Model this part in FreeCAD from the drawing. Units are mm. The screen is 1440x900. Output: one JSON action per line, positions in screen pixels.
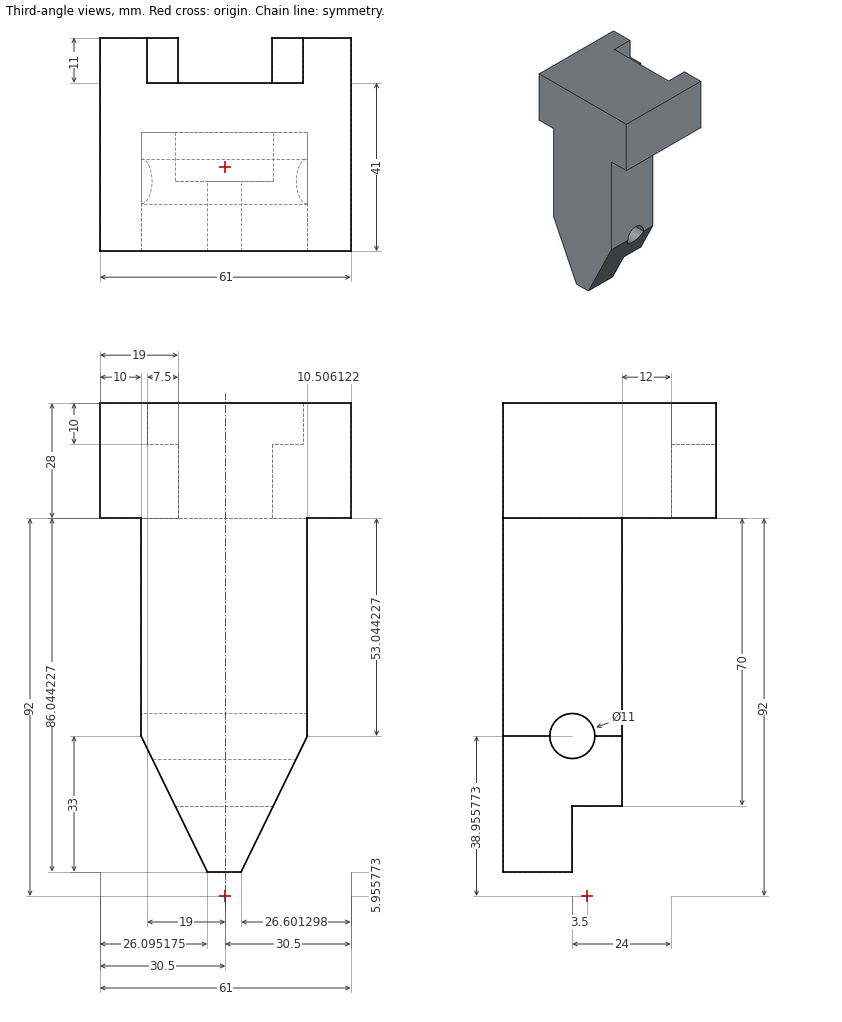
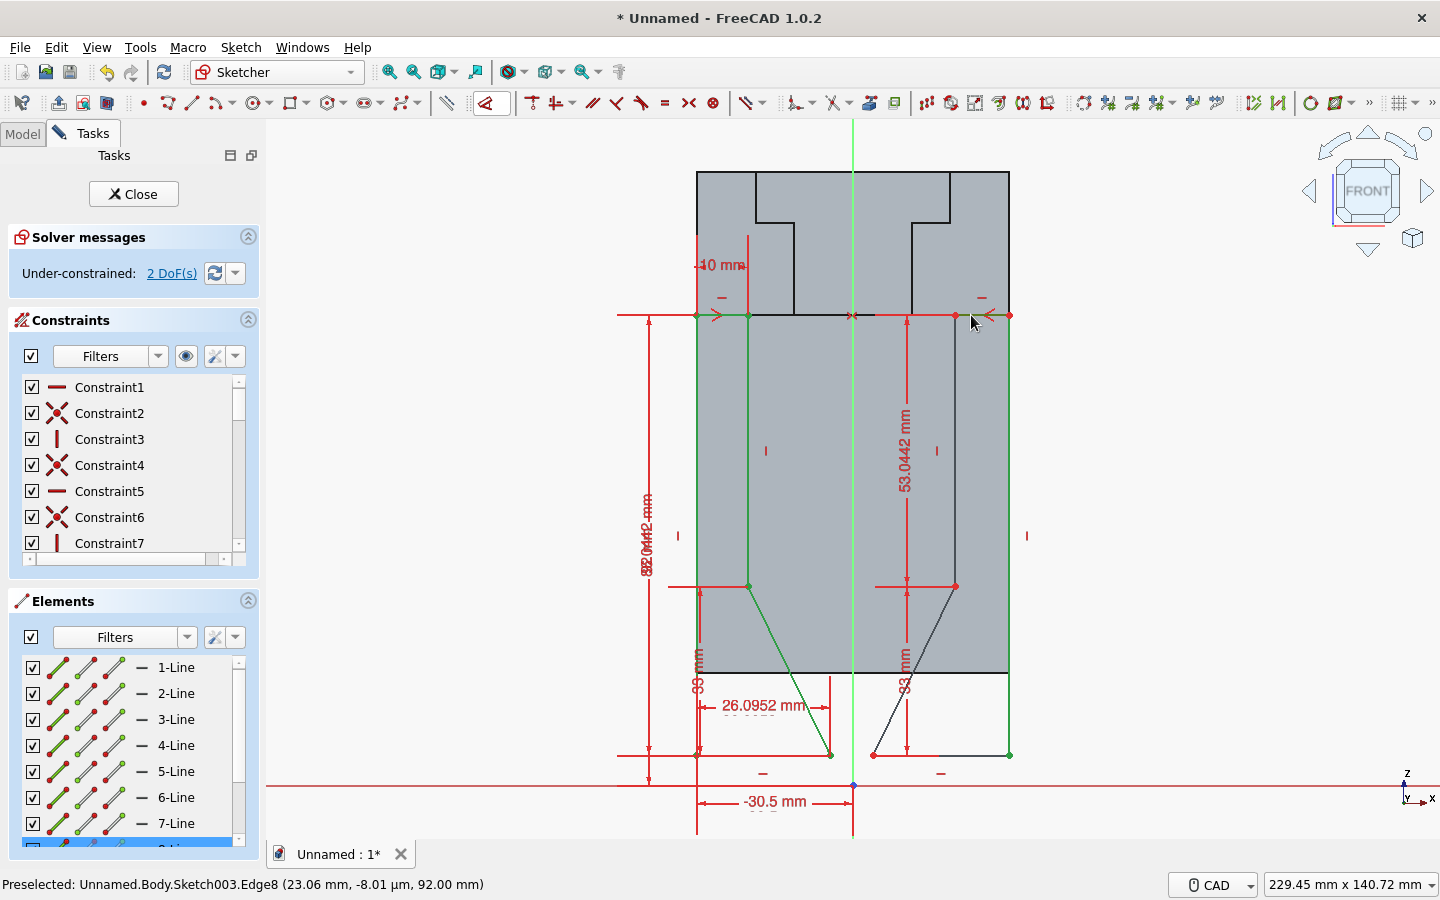
{"action": "left_click", "coordinate": [504, 104]}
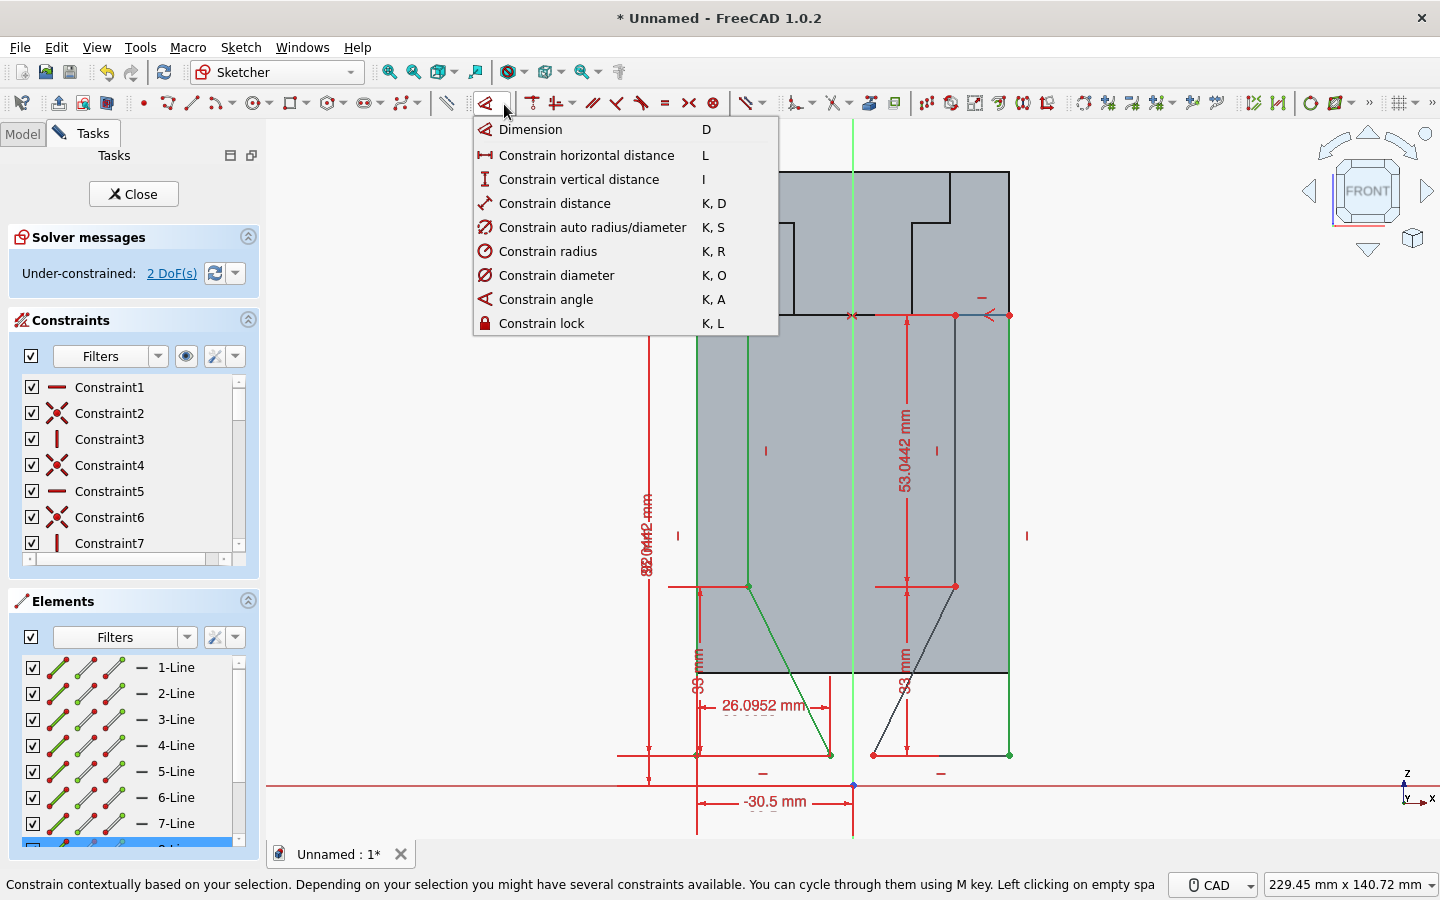
{"action": "left_click", "coordinate": [626, 155]}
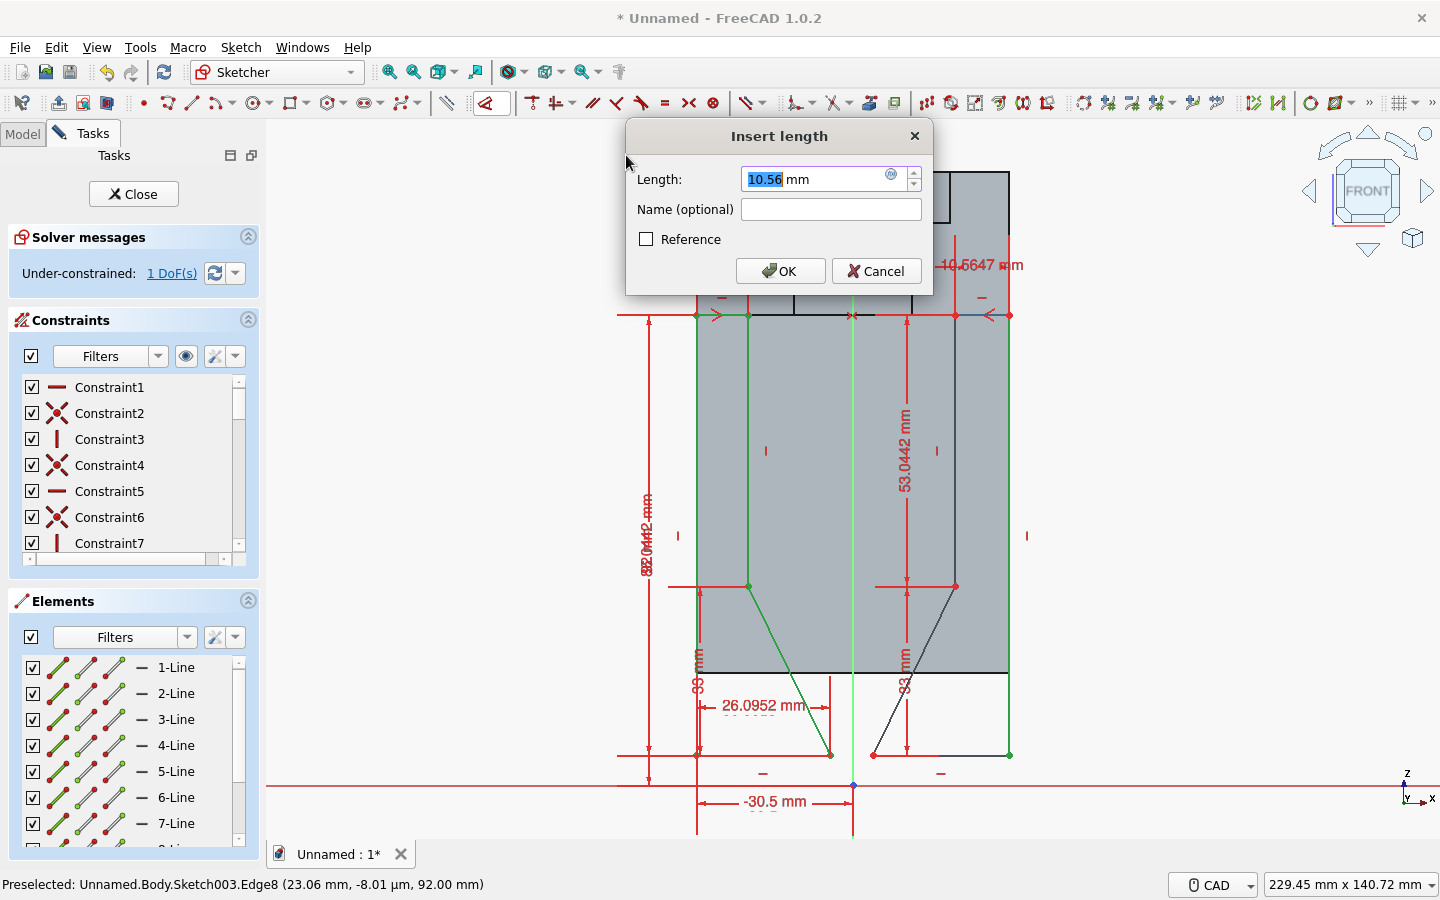
{"action": "type", "text": "10.506122"}
{"action": "key", "text": "Return"}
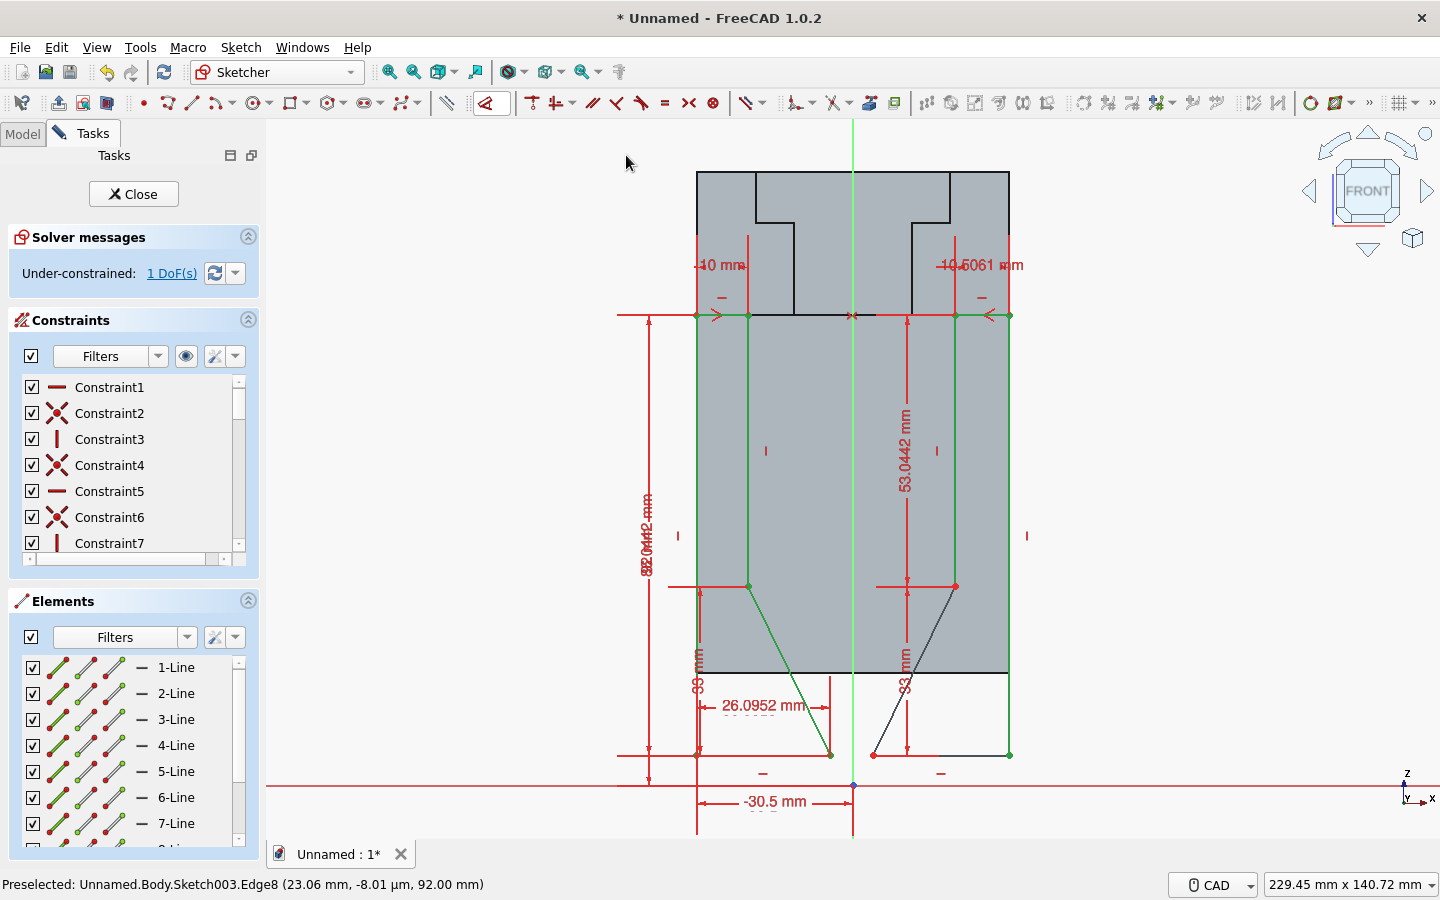
{"action": "left_click", "coordinate": [968, 756]}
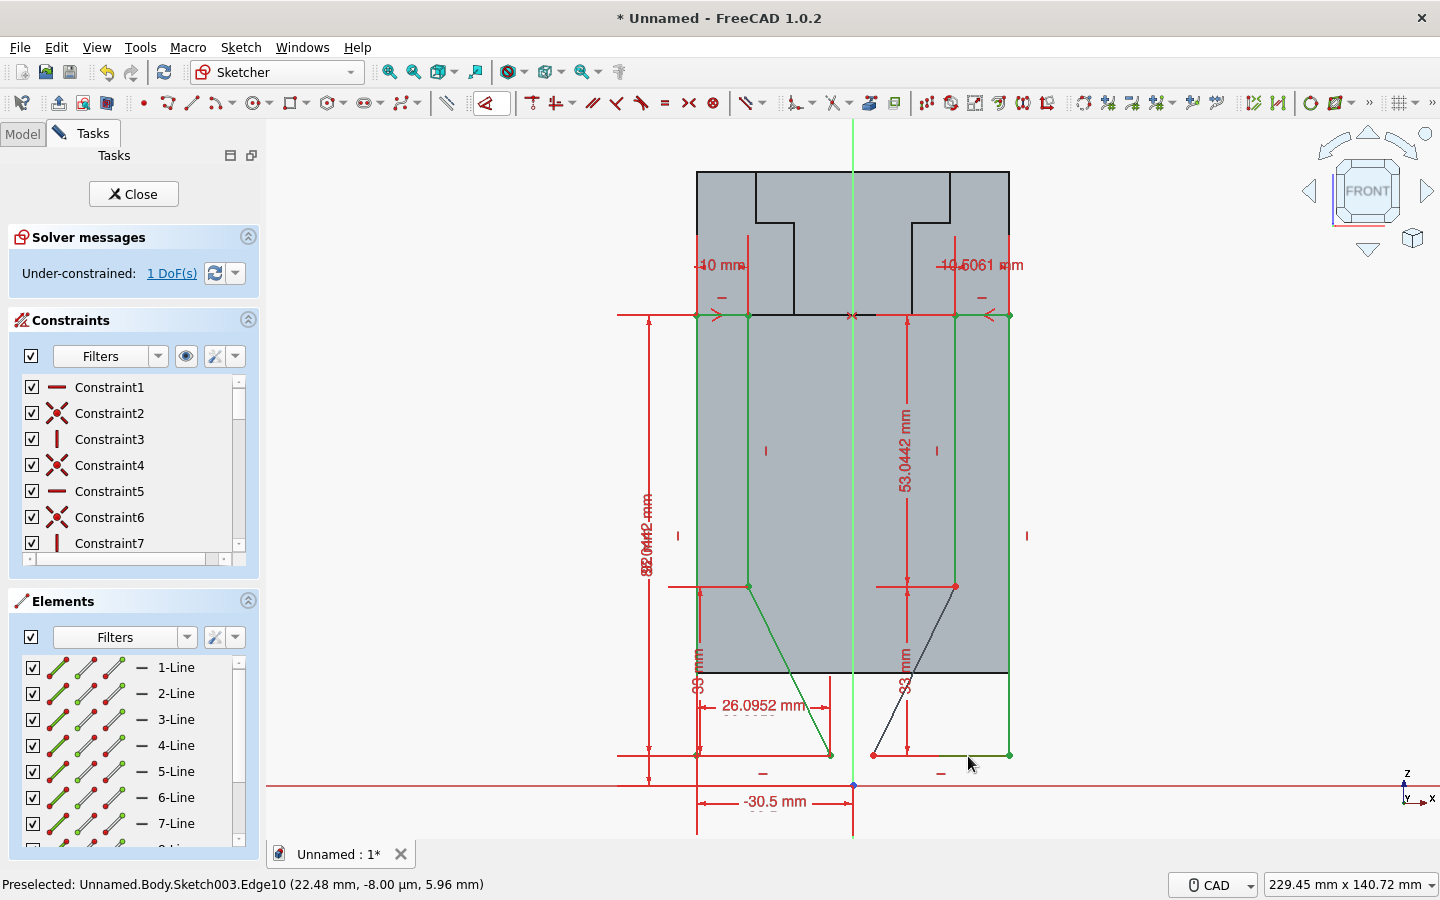
{"action": "left_click", "coordinate": [504, 104]}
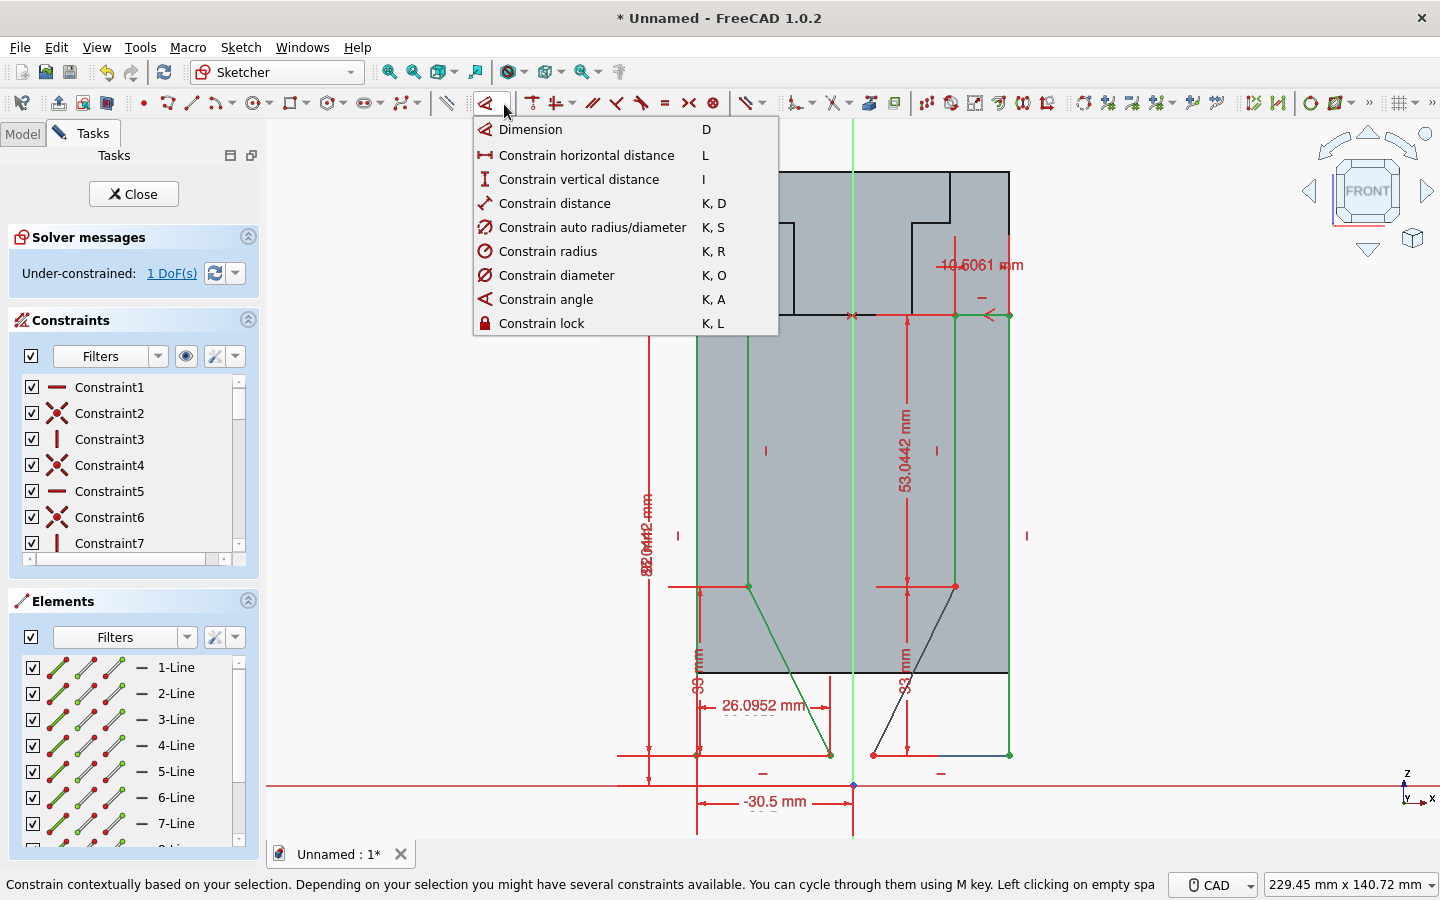
{"action": "left_click", "coordinate": [626, 155]}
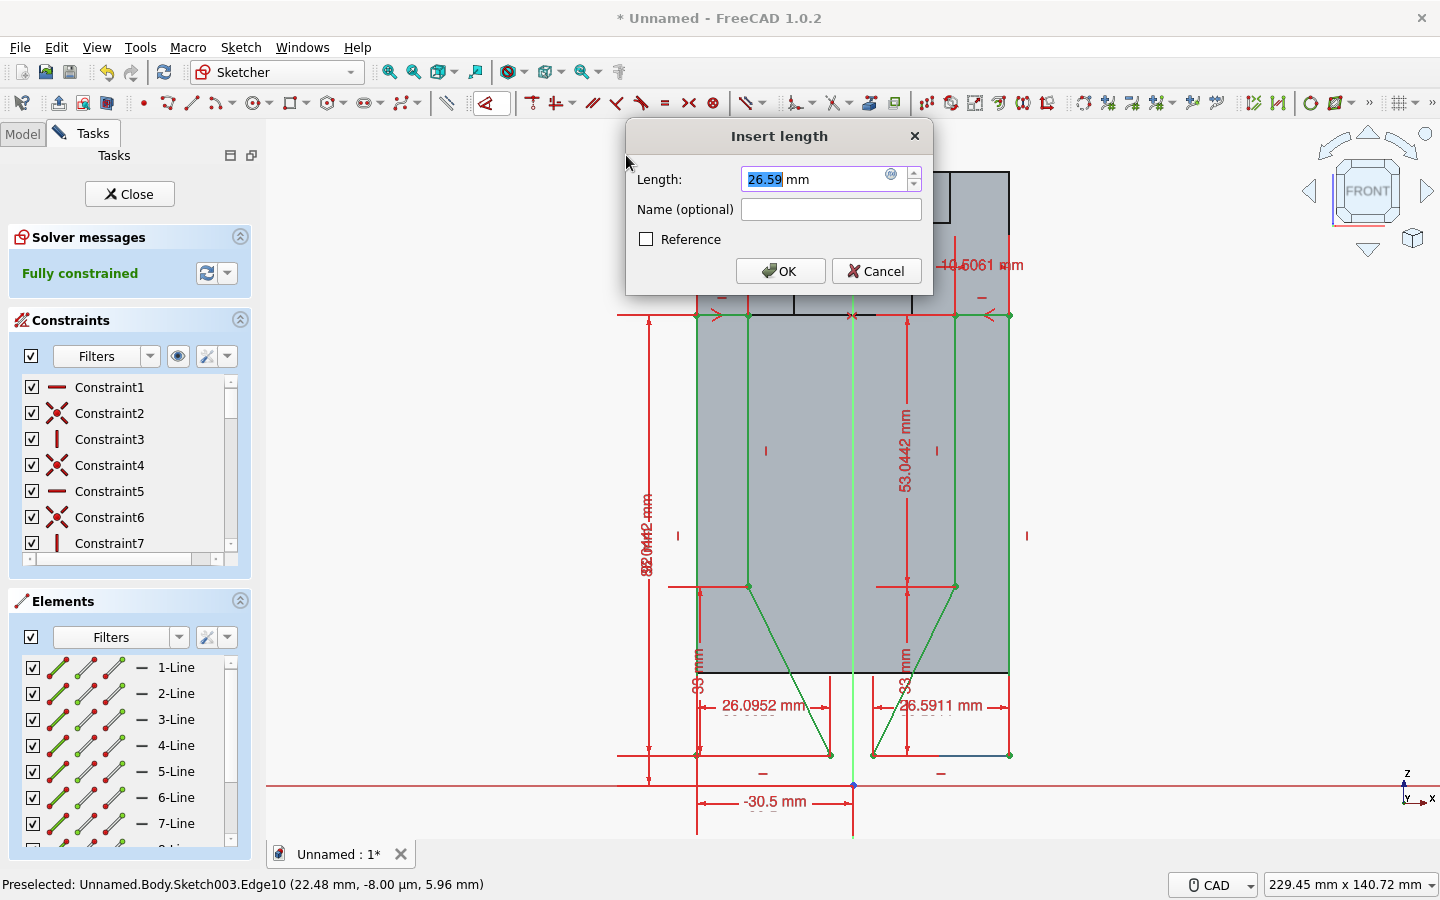
{"action": "type", "text": "26.601298"}
{"action": "key", "text": "Return"}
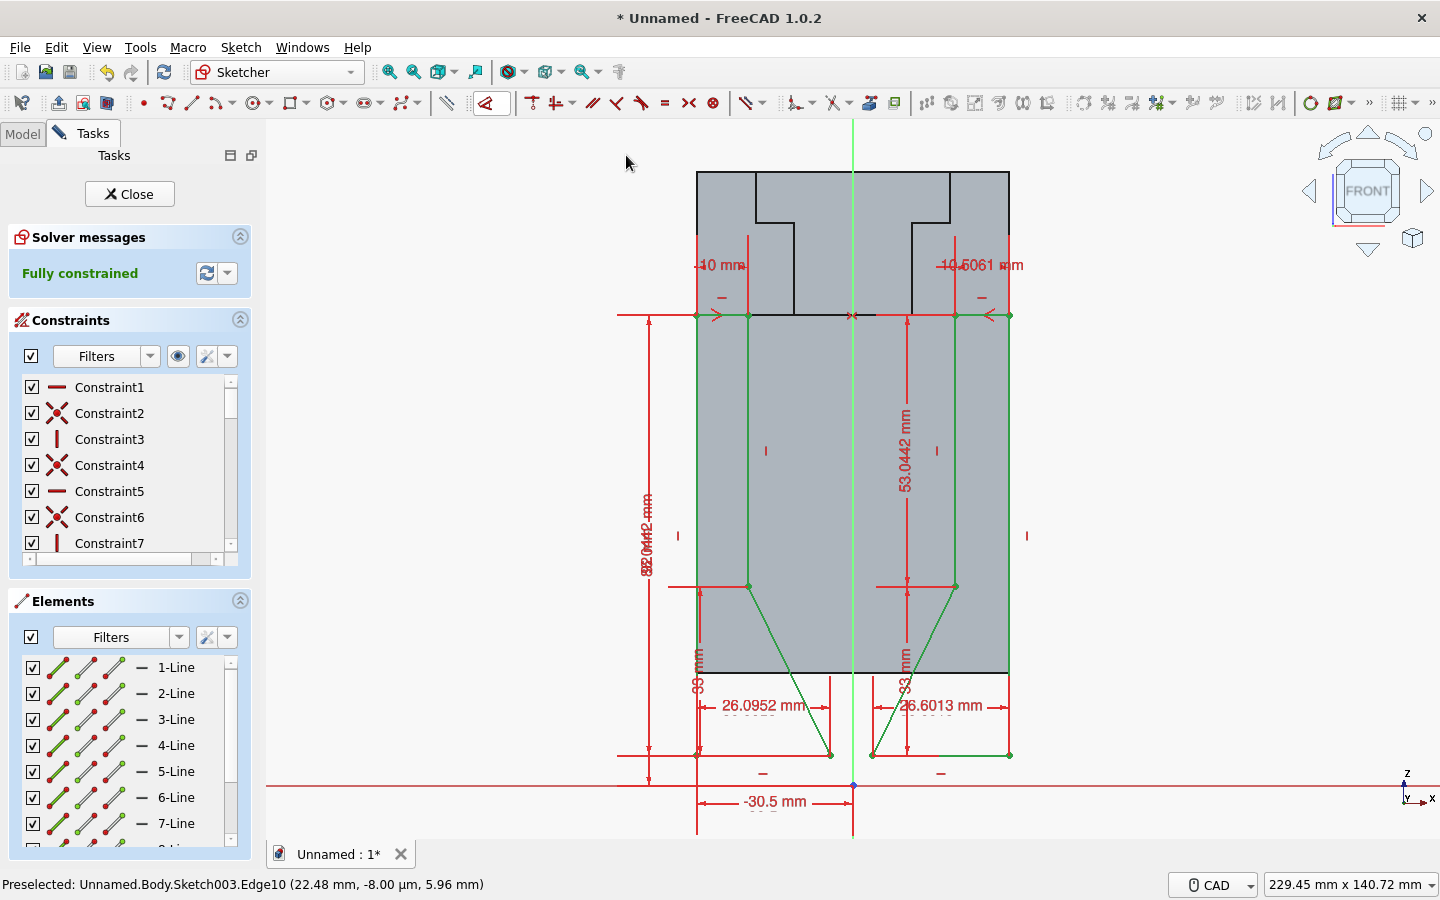
{"action": "left_click", "coordinate": [130, 194]}